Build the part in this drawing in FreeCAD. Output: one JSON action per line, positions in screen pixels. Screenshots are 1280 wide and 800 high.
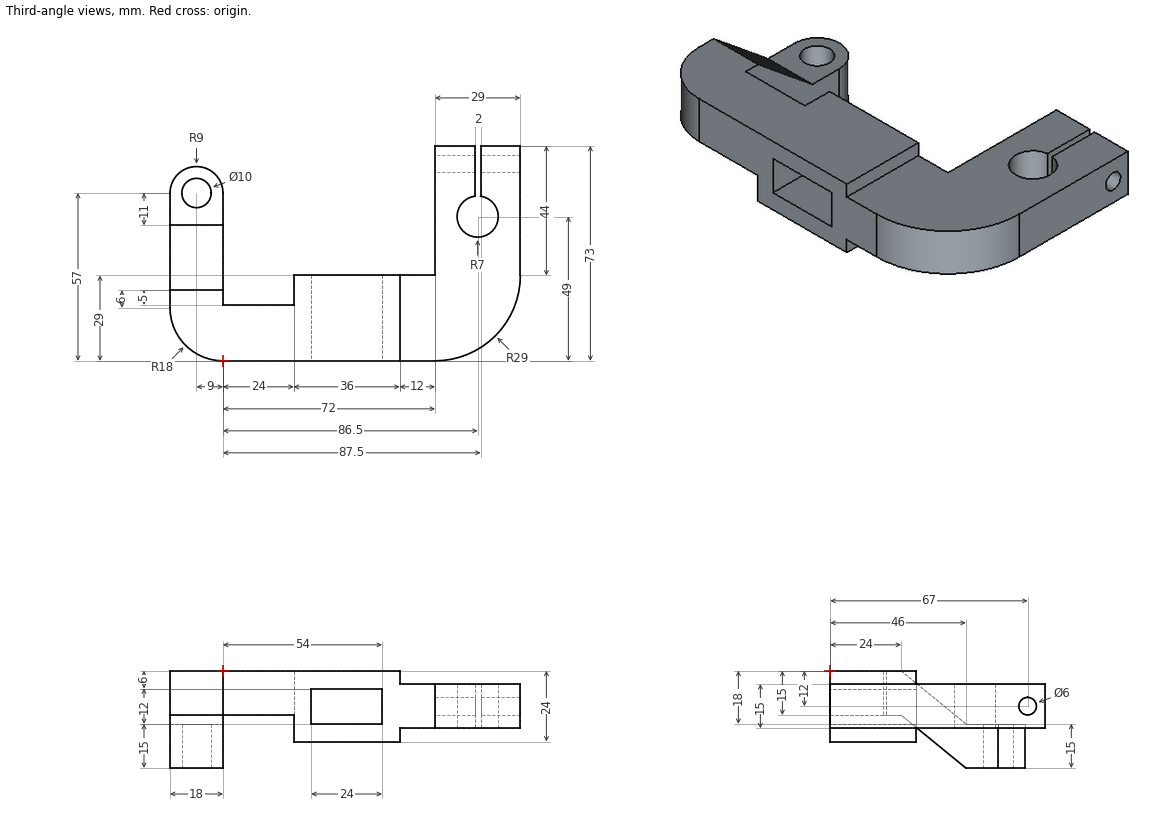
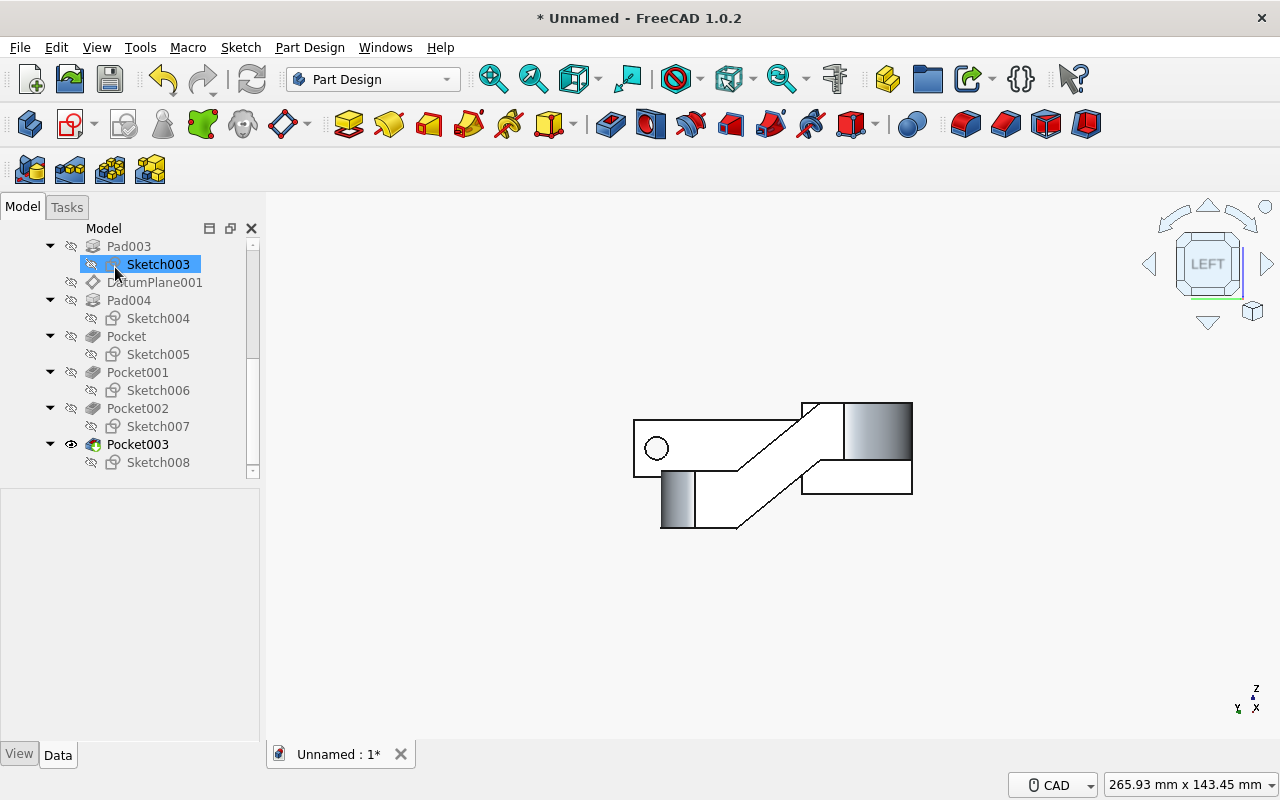
{"action": "key", "text": "0"}